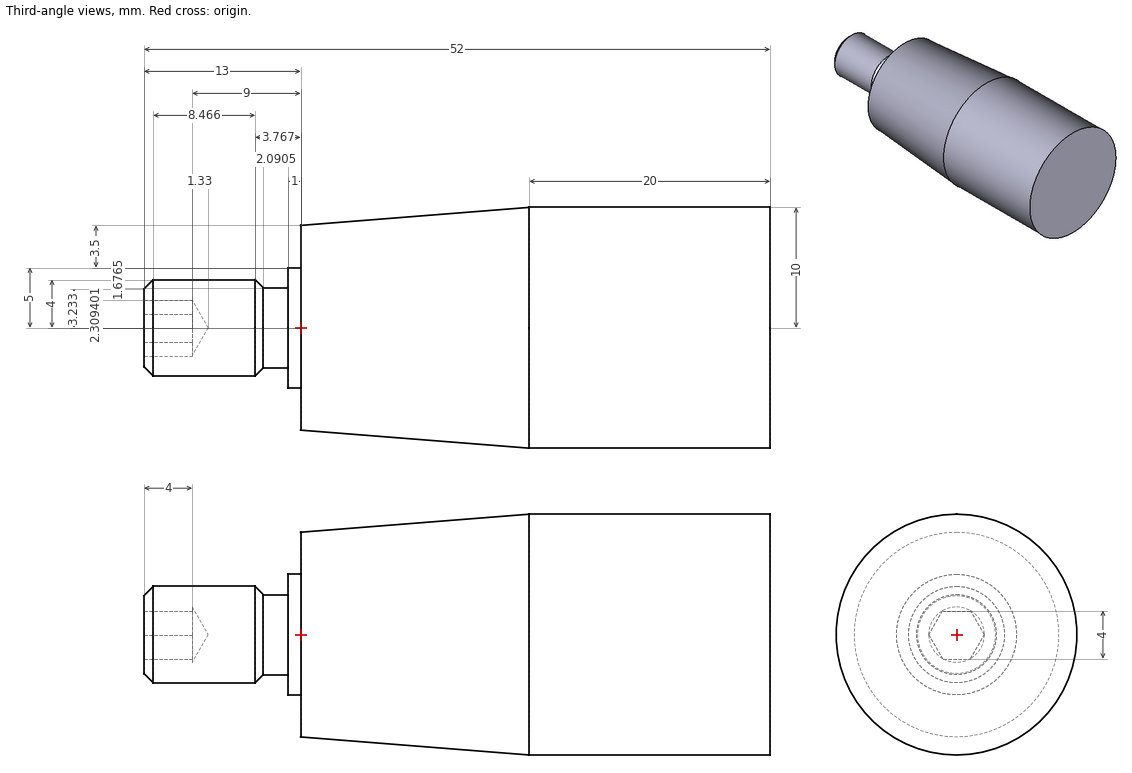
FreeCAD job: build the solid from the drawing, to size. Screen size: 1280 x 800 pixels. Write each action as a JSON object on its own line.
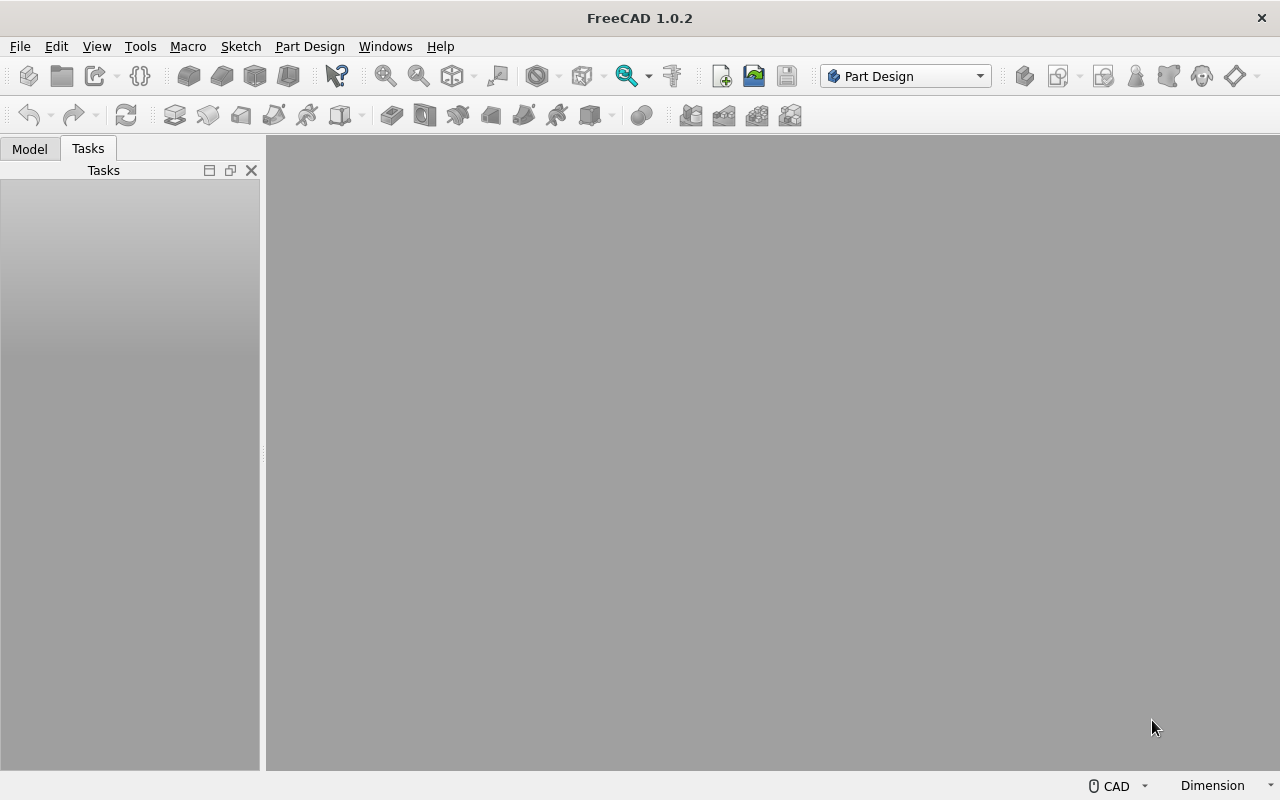
{"action": "left_click", "coordinate": [721, 76]}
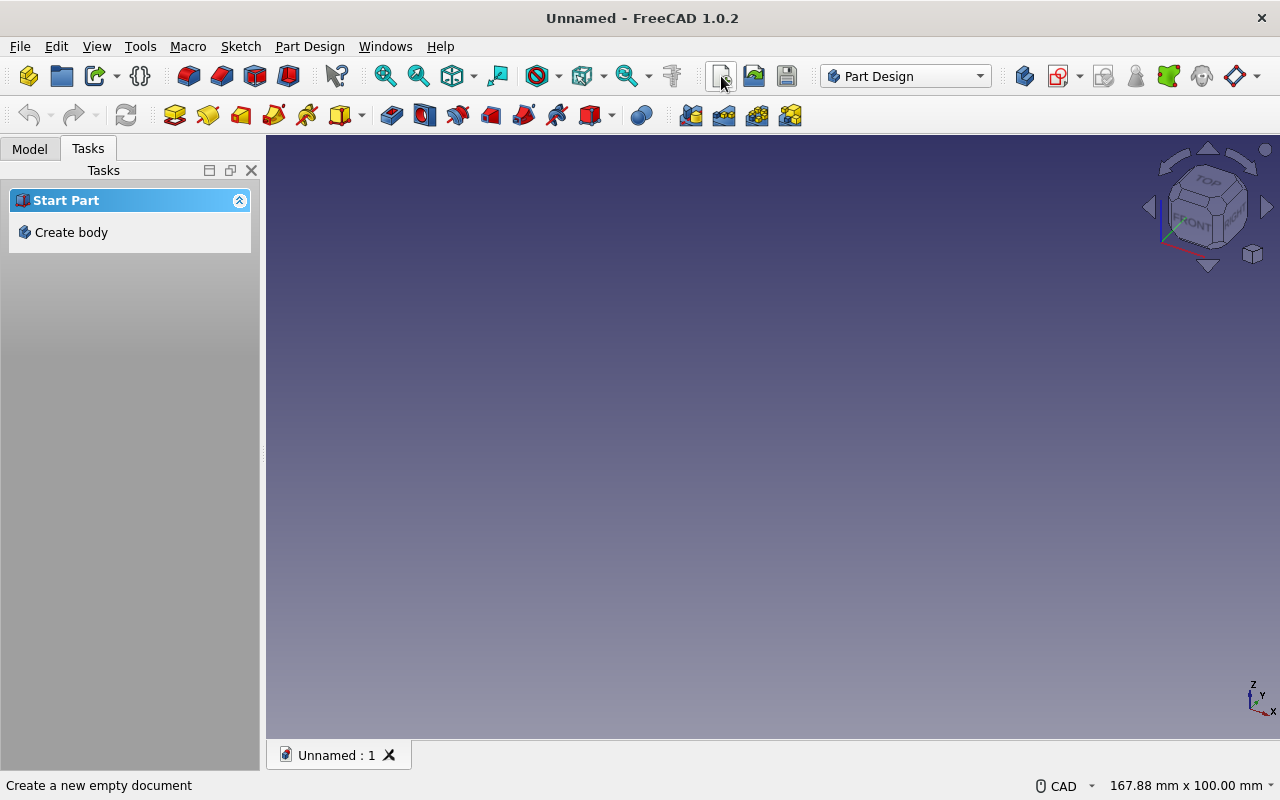
{"action": "left_click", "coordinate": [1058, 76]}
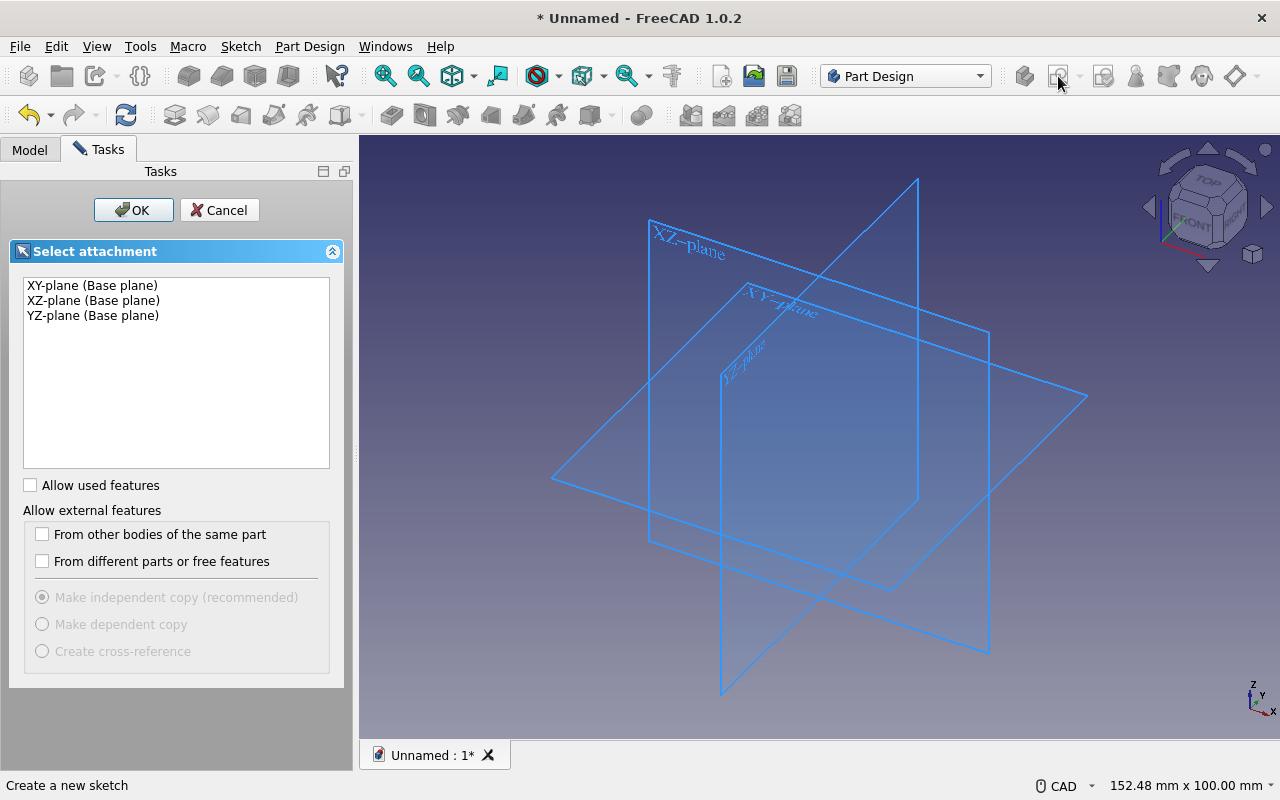
{"action": "left_click", "coordinate": [84, 286]}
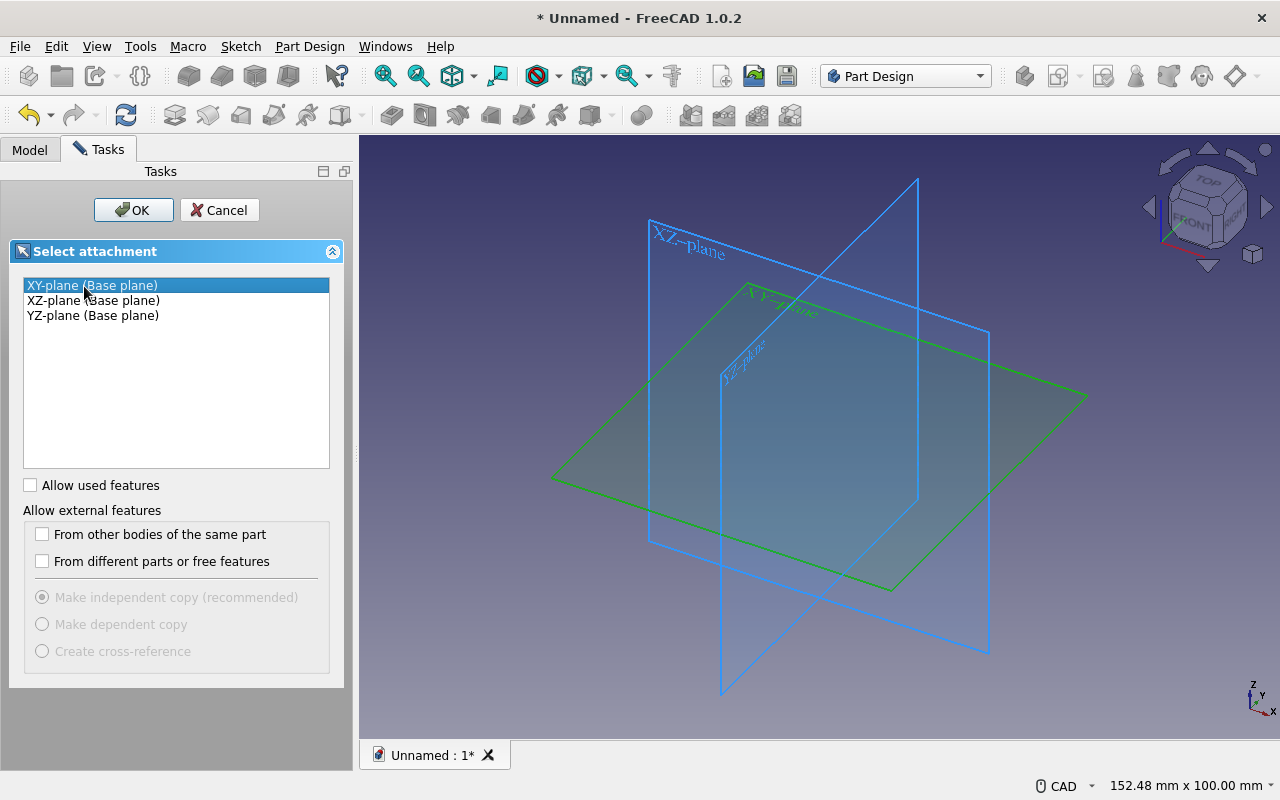
{"action": "left_click", "coordinate": [134, 210]}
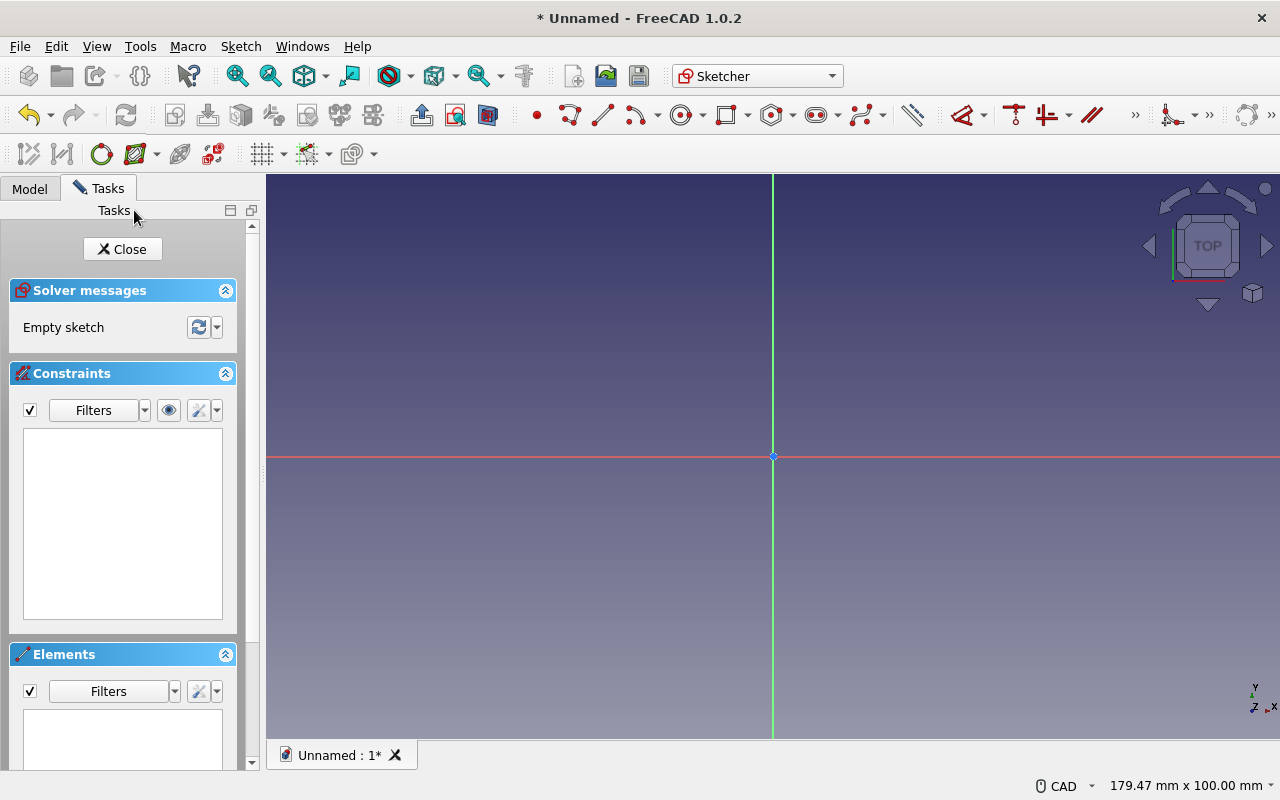
{"action": "scroll", "coordinate": [1019, 394], "scroll_direction": "up", "scroll_amount": 3}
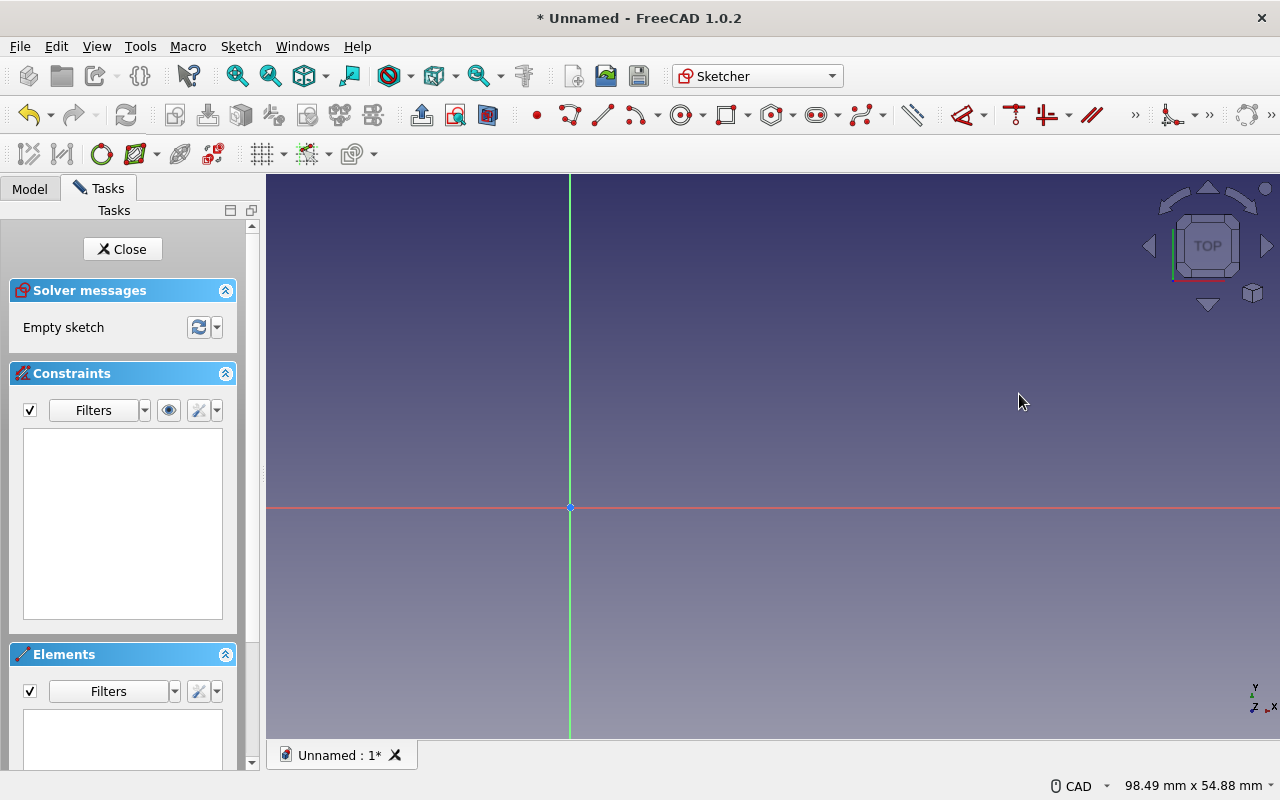
{"action": "key", "text": "g m"}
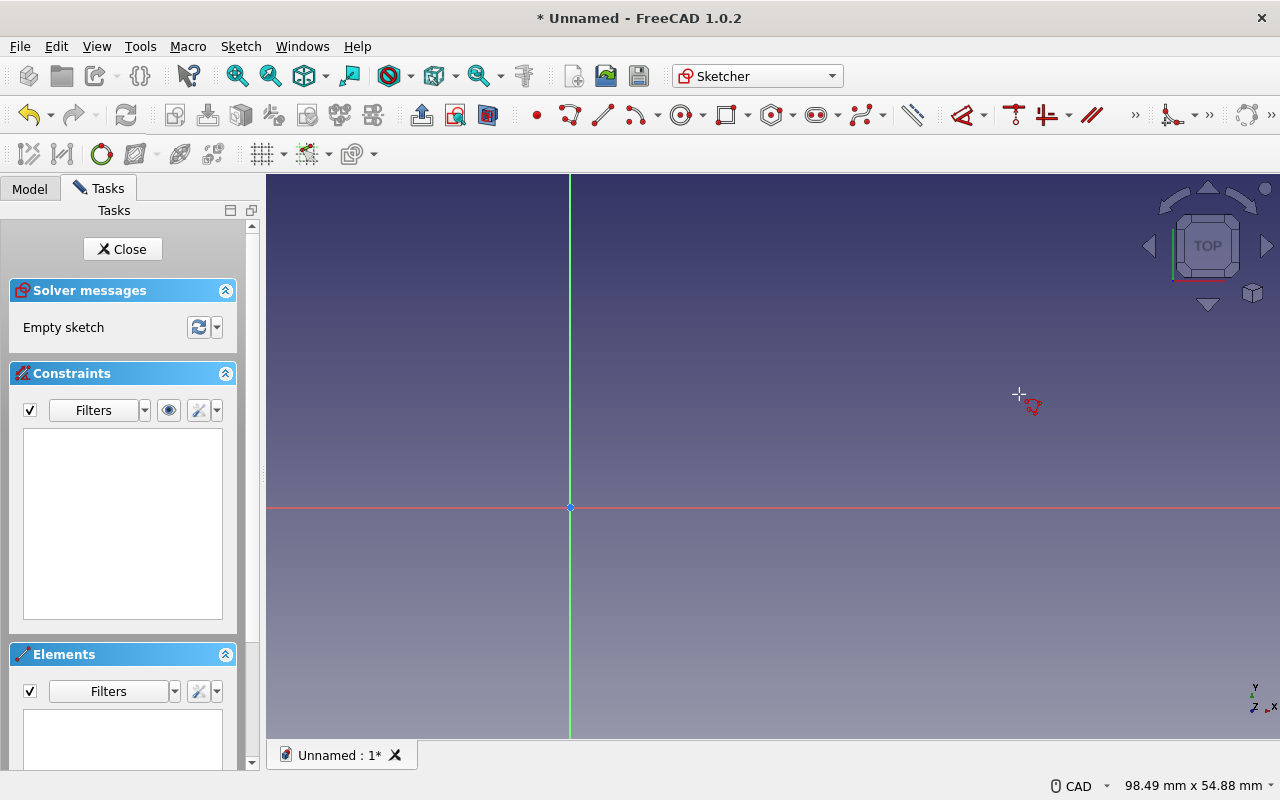
{"action": "scroll", "coordinate": [560, 473], "scroll_direction": "up", "scroll_amount": 3}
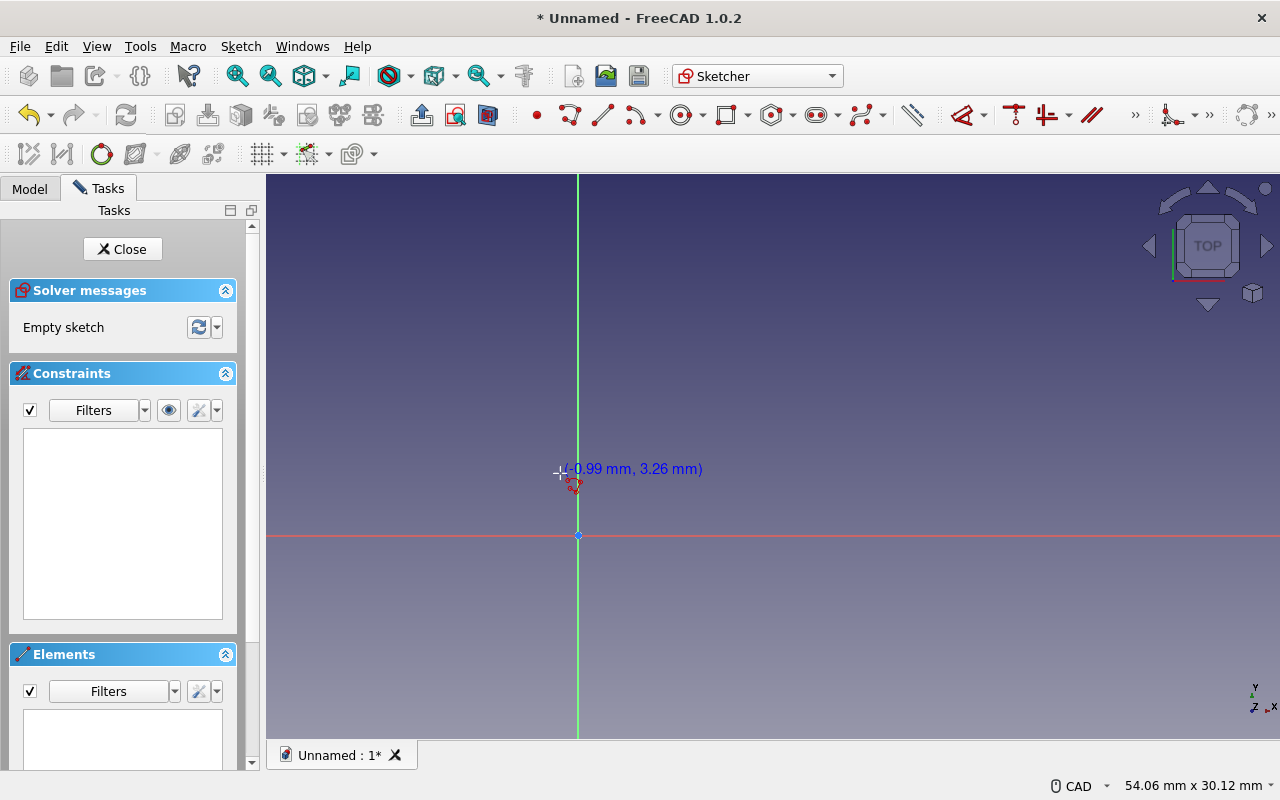
{"action": "left_click", "coordinate": [559, 473]}
{"action": "left_click", "coordinate": [520, 473]}
{"action": "left_click", "coordinate": [508, 461]}
{"action": "left_click", "coordinate": [349, 461]}
{"action": "left_click", "coordinate": [334, 475]}
{"action": "left_click", "coordinate": [334, 536]}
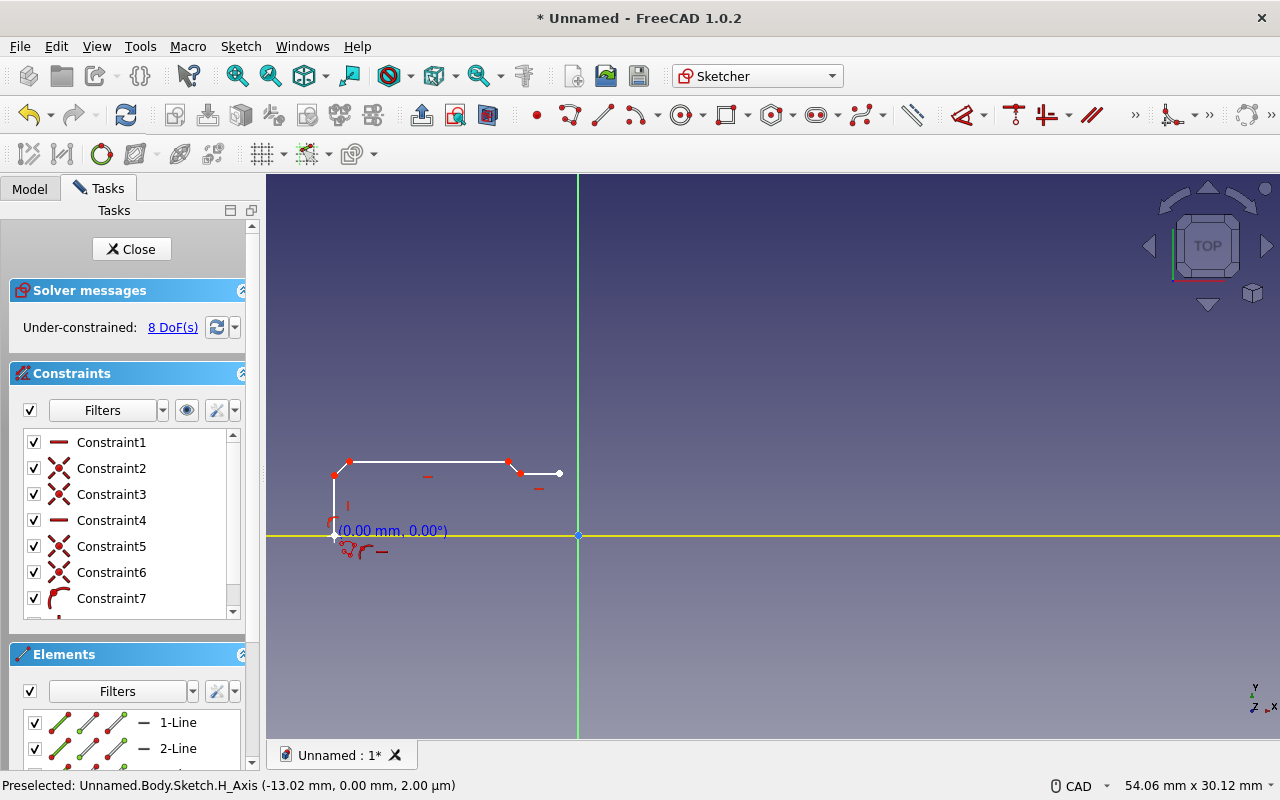
{"action": "scroll", "coordinate": [561, 474], "scroll_direction": "down", "scroll_amount": 3}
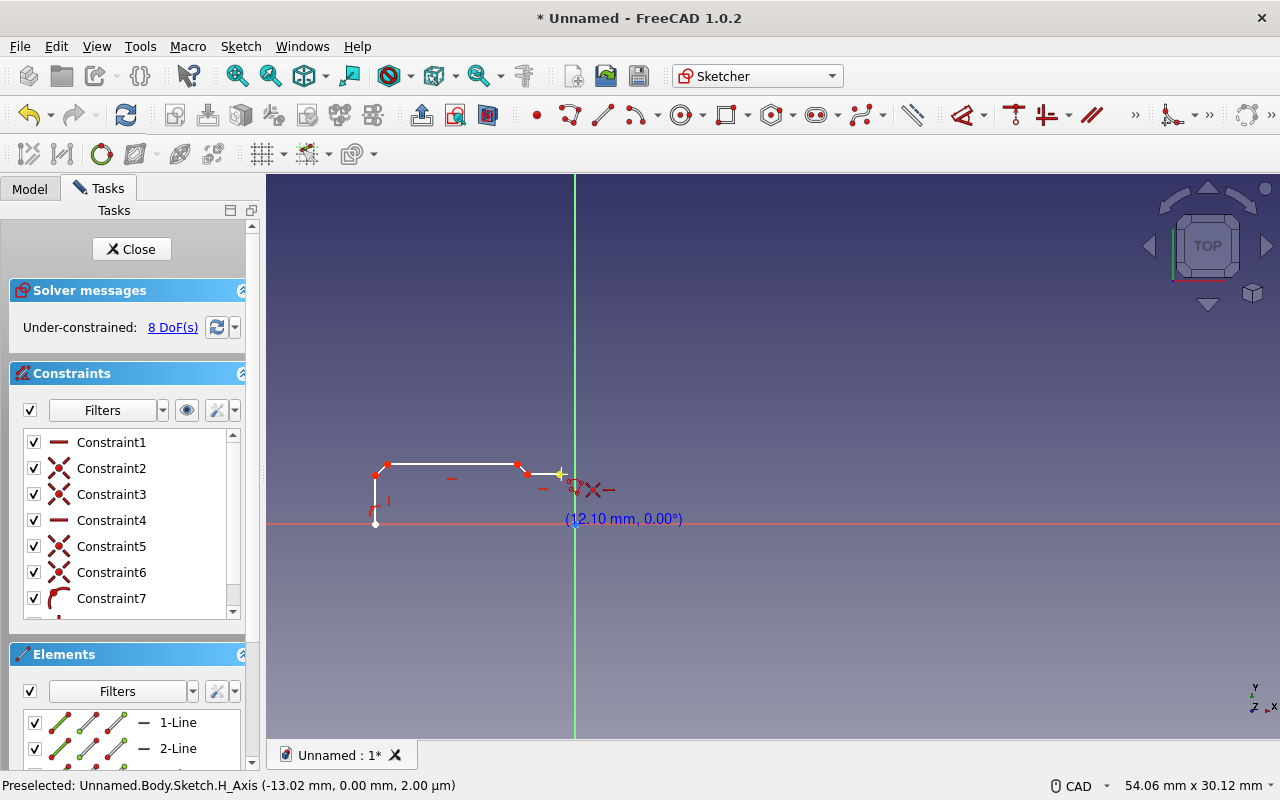
{"action": "left_click", "coordinate": [972, 499]}
{"action": "left_click", "coordinate": [972, 405]}
{"action": "left_click", "coordinate": [766, 405]}
{"action": "left_click", "coordinate": [571, 421]}
{"action": "left_click", "coordinate": [580, 457]}